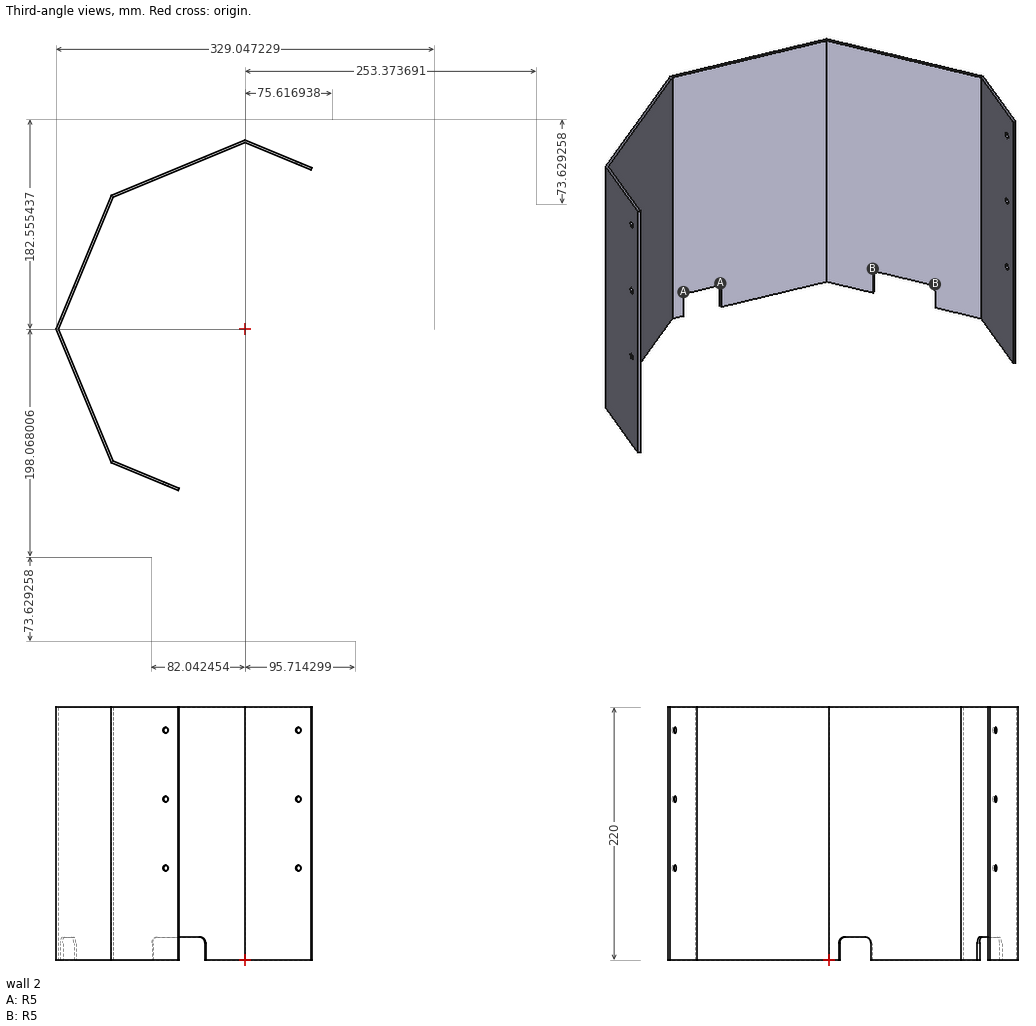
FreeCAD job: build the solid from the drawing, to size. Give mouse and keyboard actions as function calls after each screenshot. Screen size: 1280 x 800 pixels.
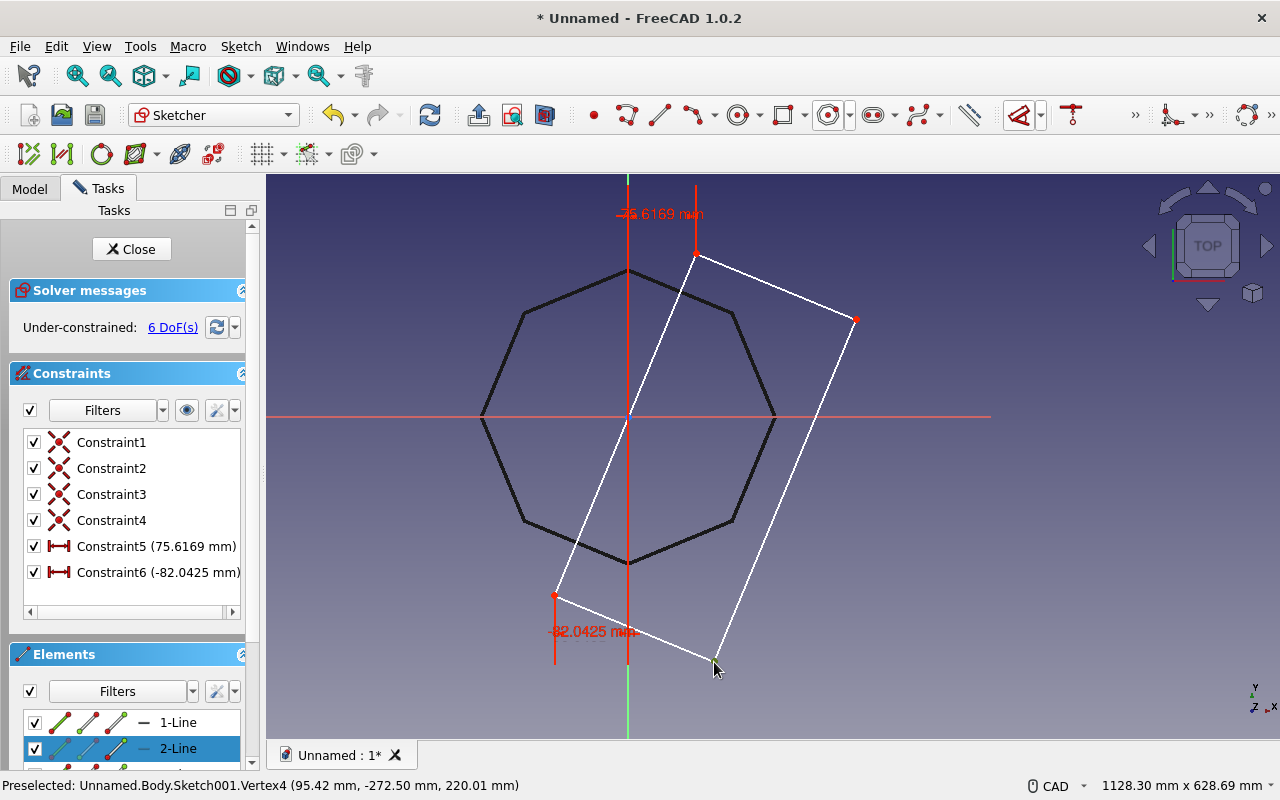
click(1040, 116)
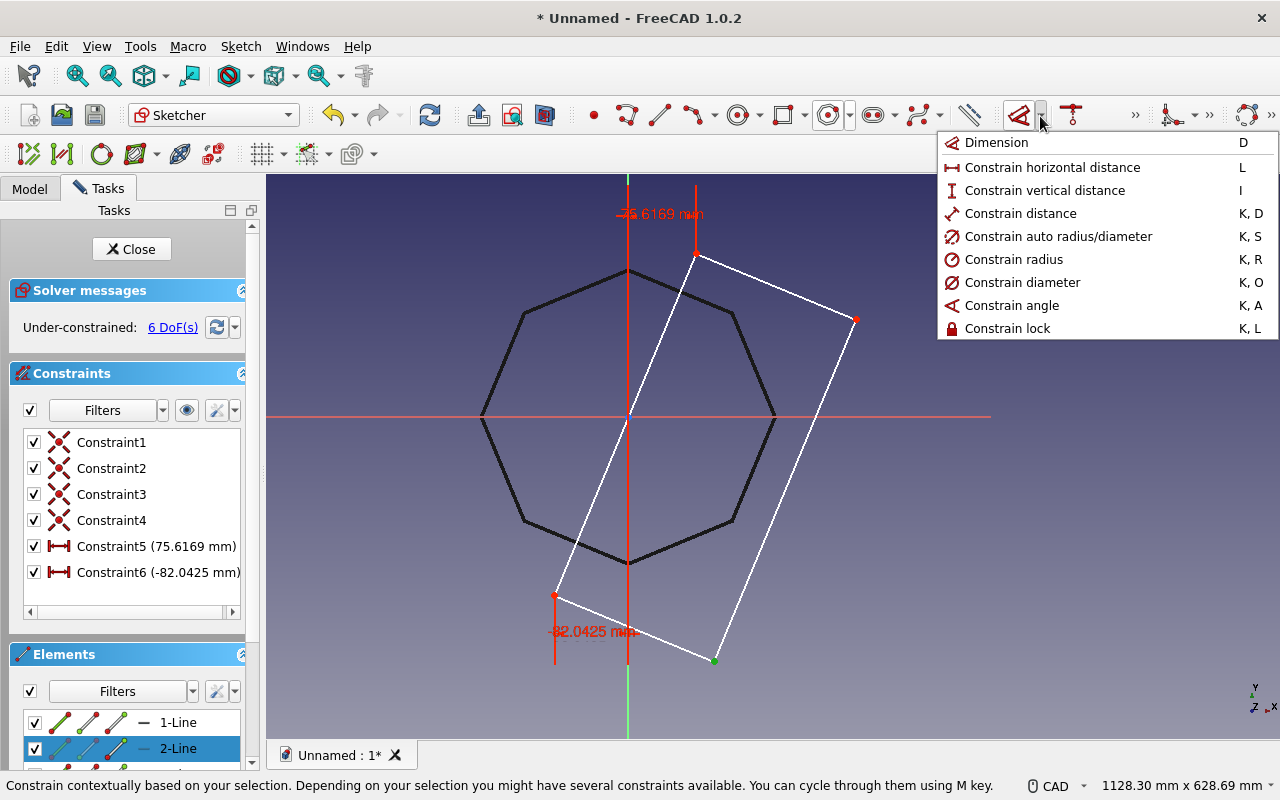
click(1108, 168)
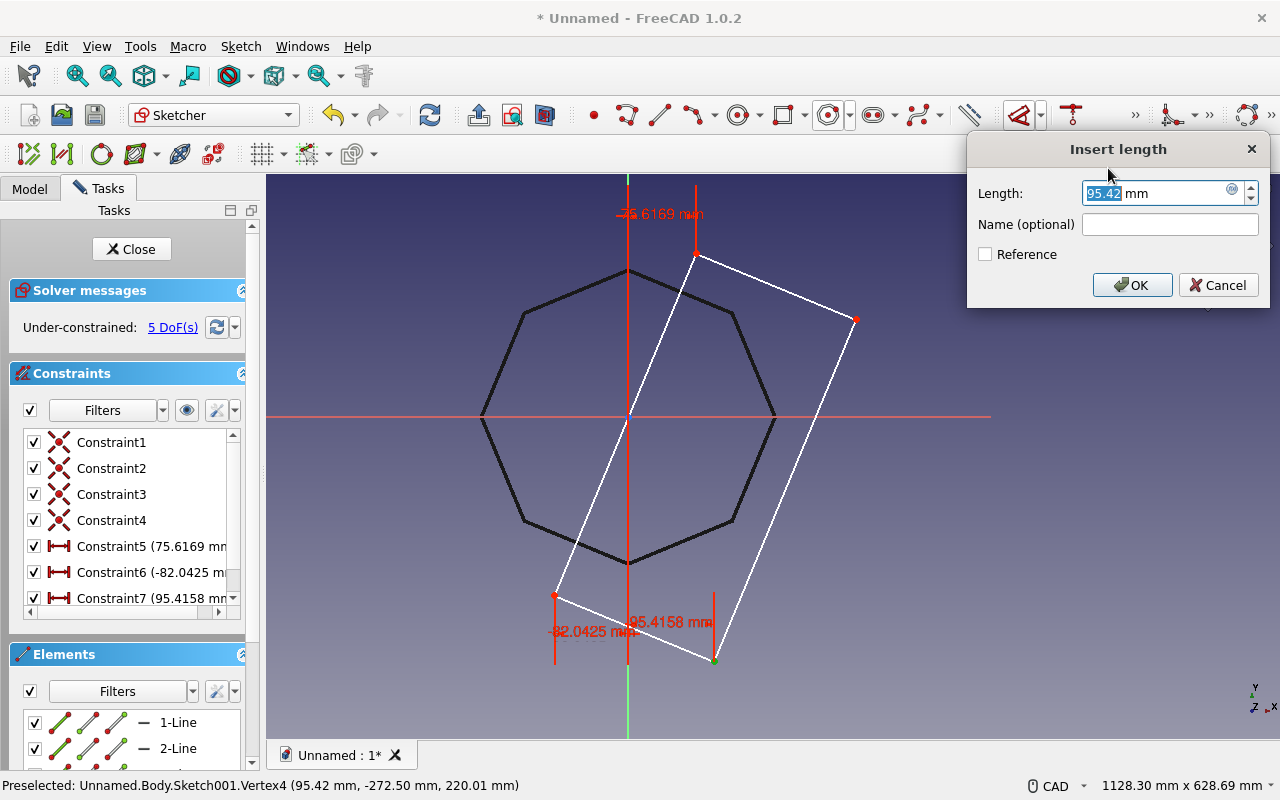
text(95.714299)
key(Return)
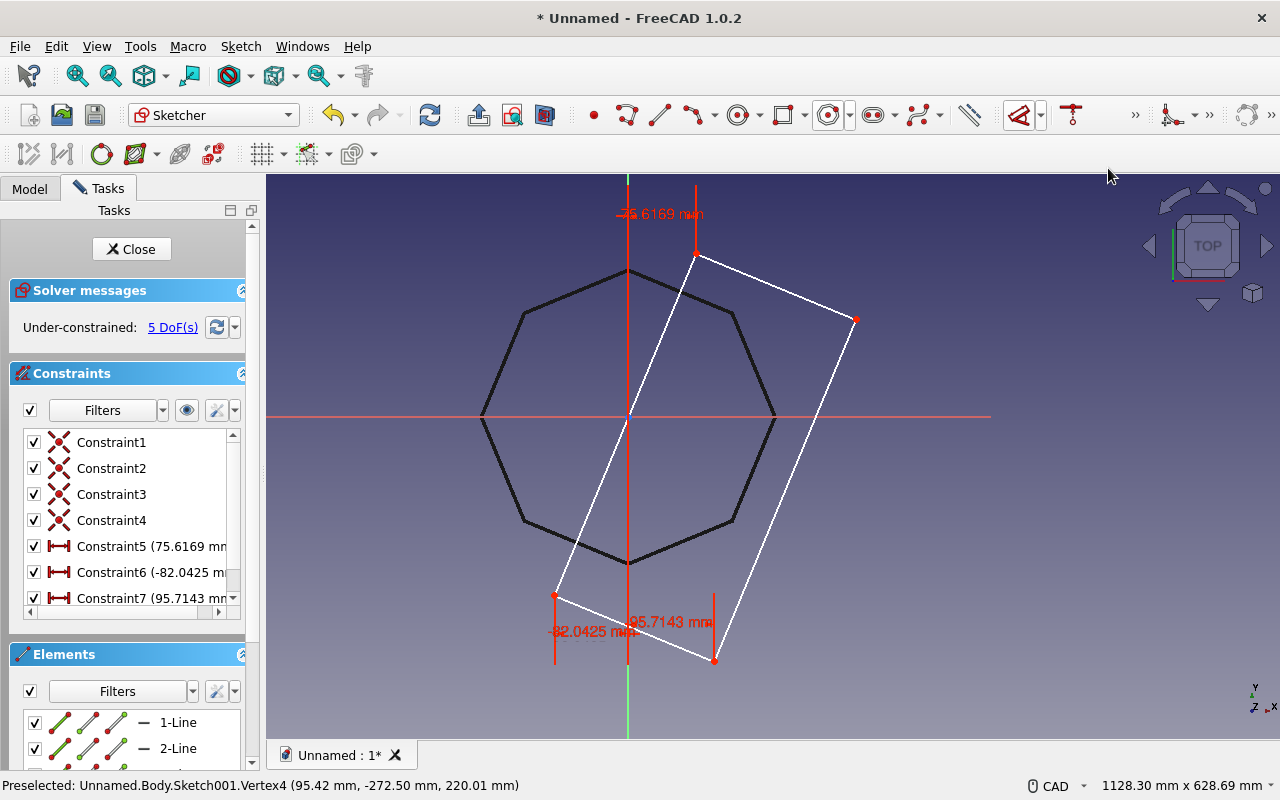
click(602, 616)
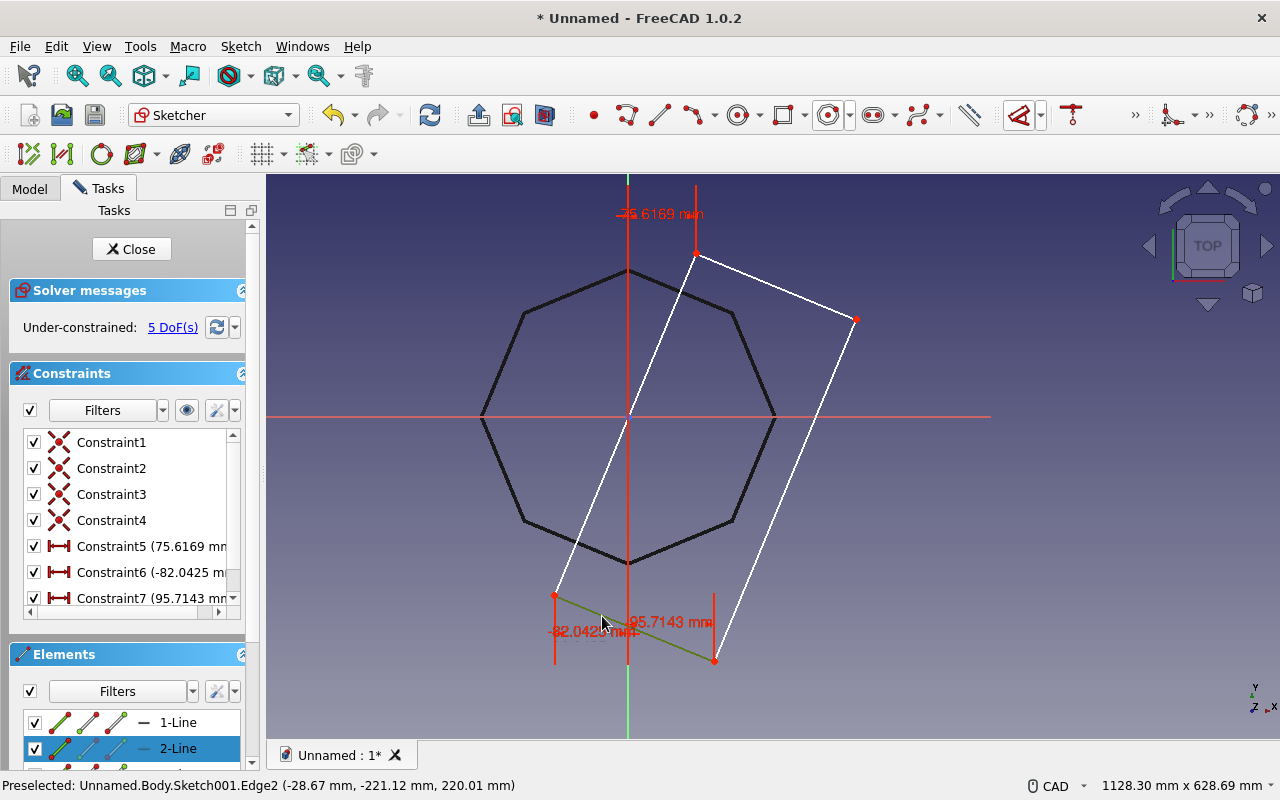
key(i)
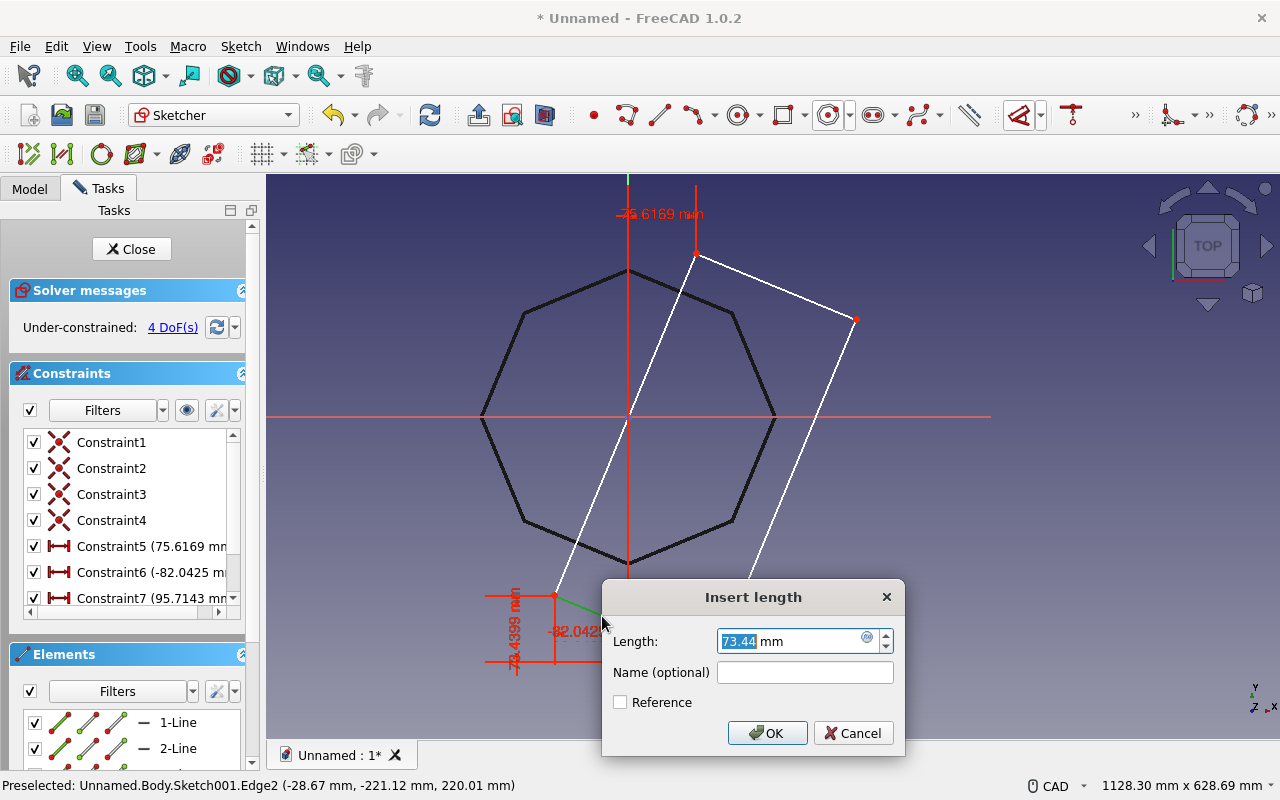
text(73.629258)
key(Return)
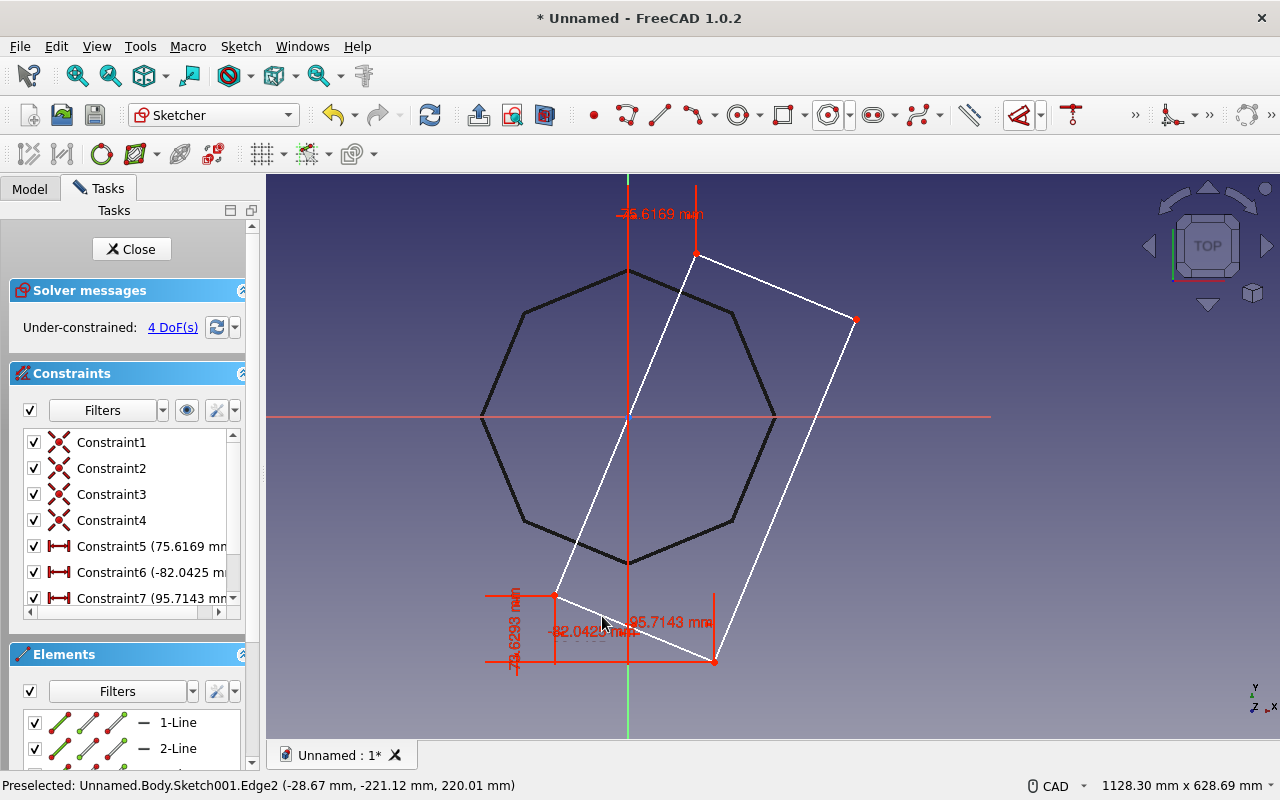
click(808, 300)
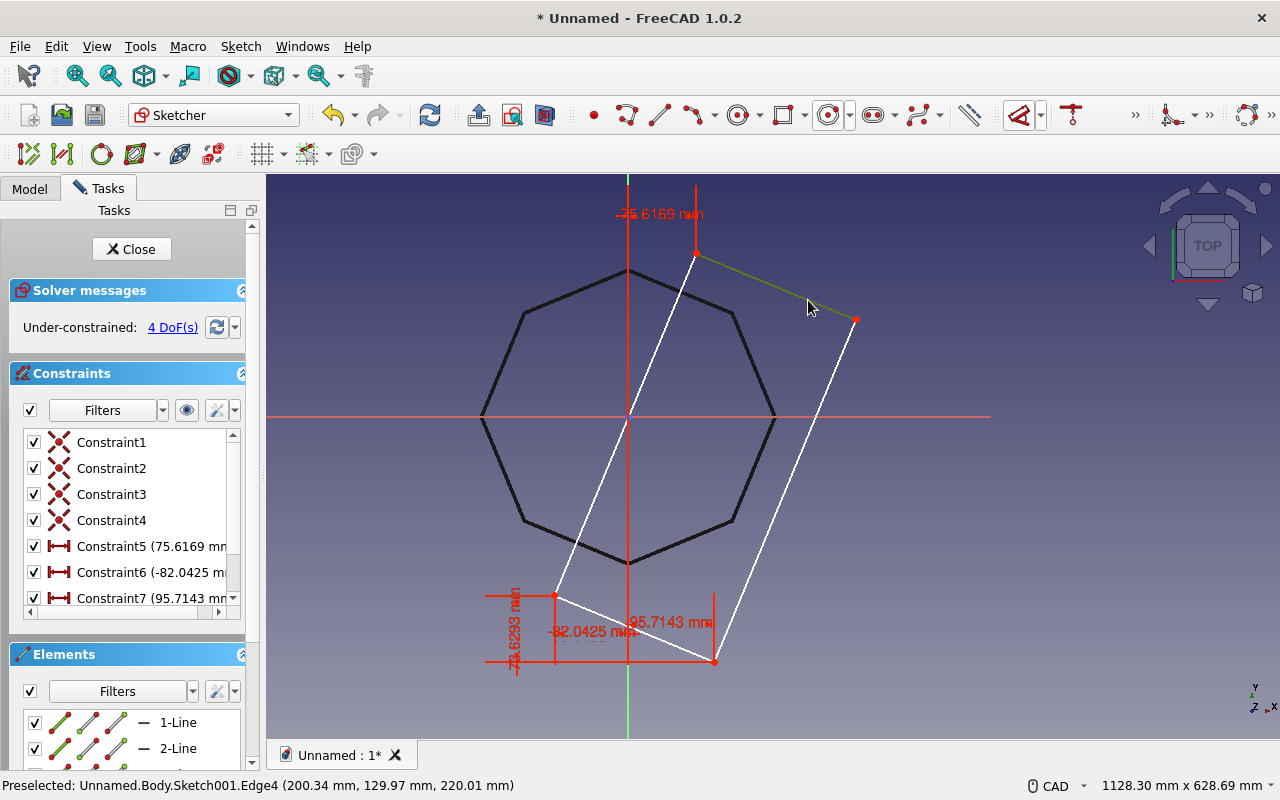
click(1040, 116)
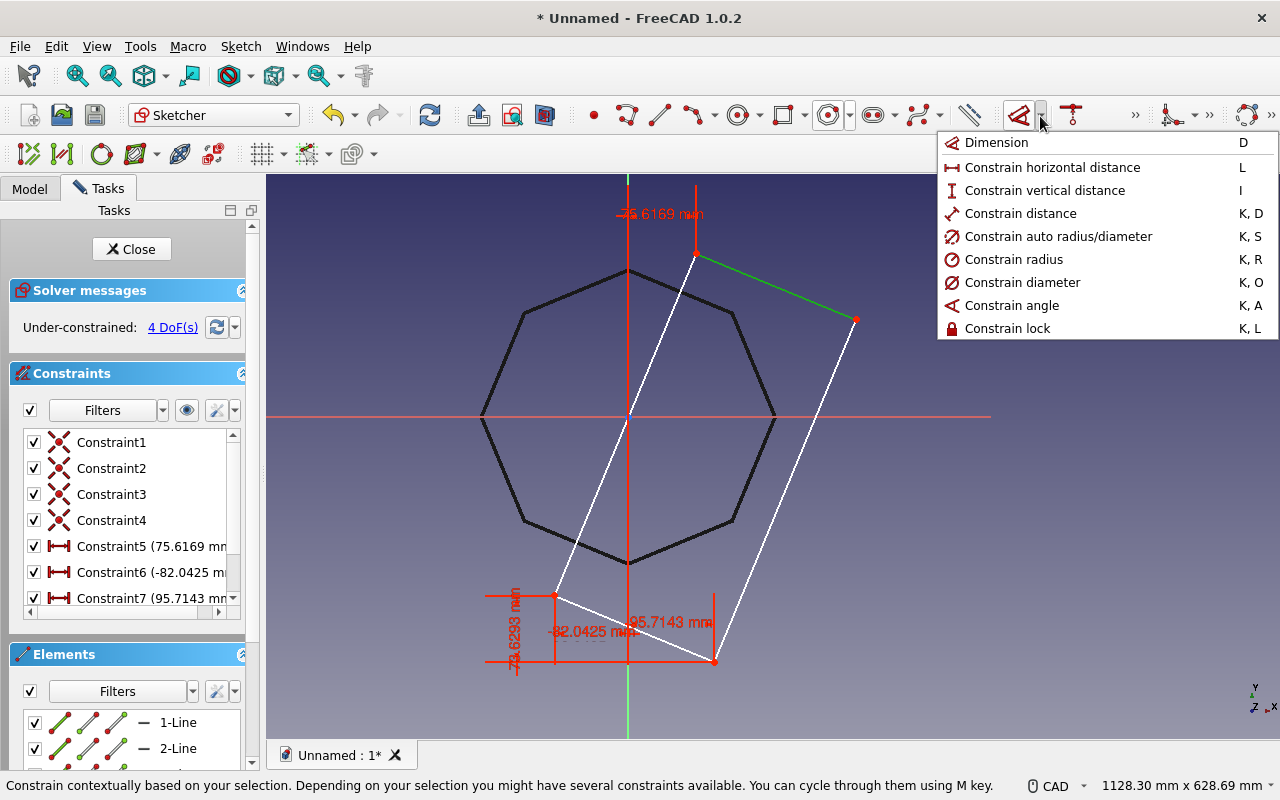
click(1108, 190)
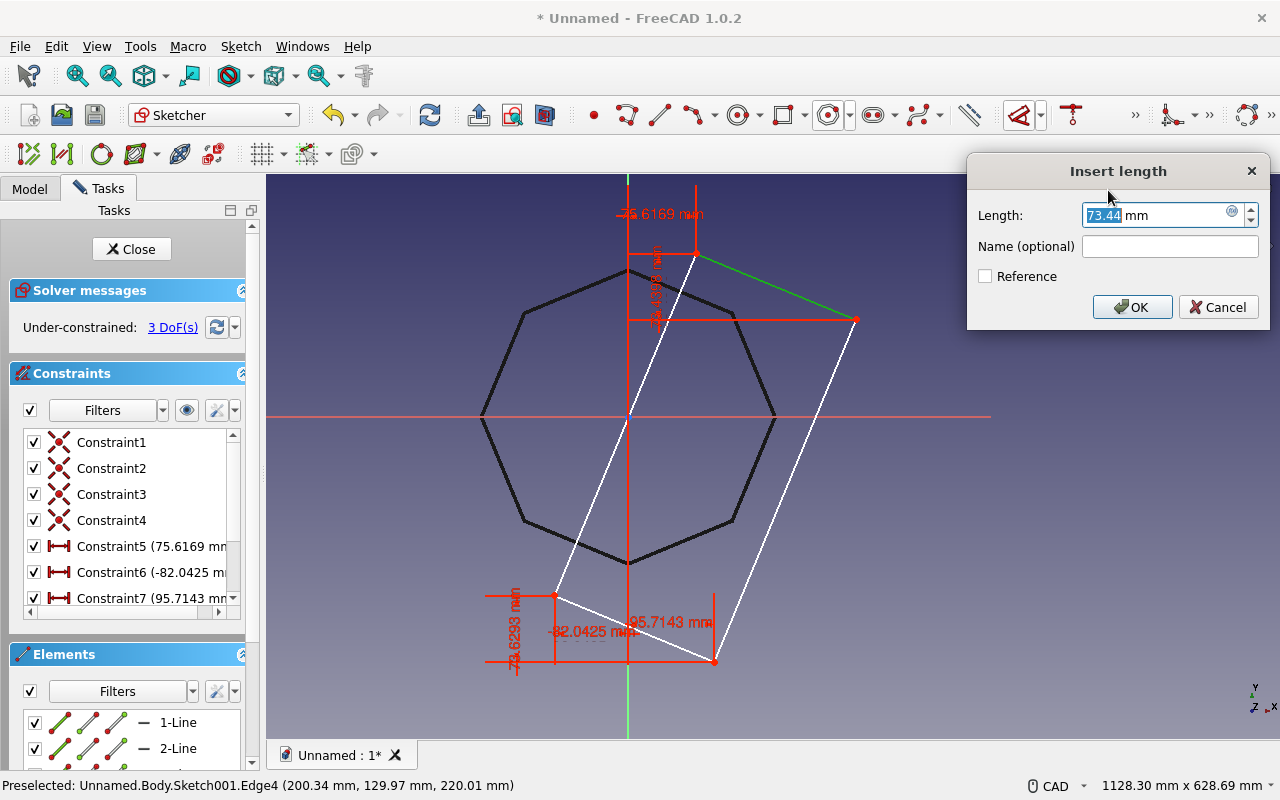
text(73.629258)
key(Return)